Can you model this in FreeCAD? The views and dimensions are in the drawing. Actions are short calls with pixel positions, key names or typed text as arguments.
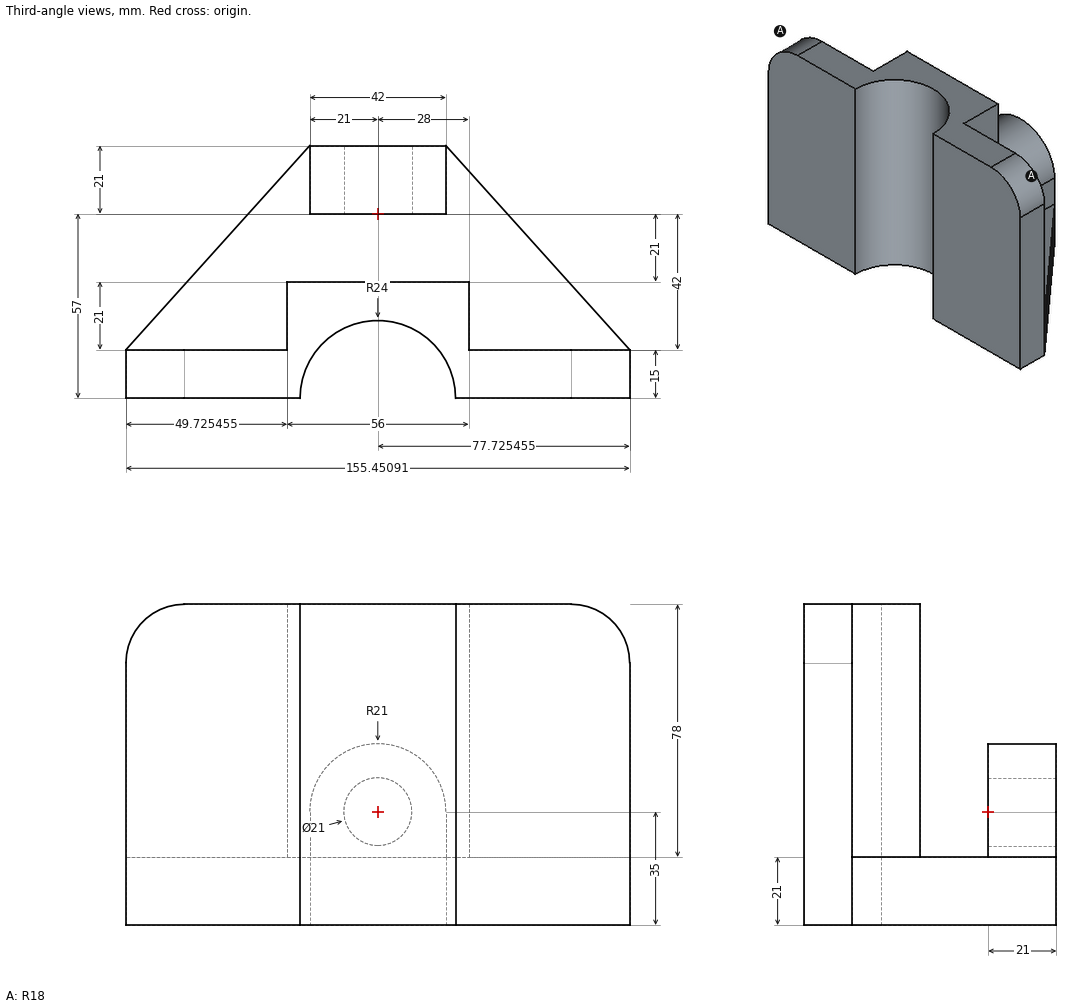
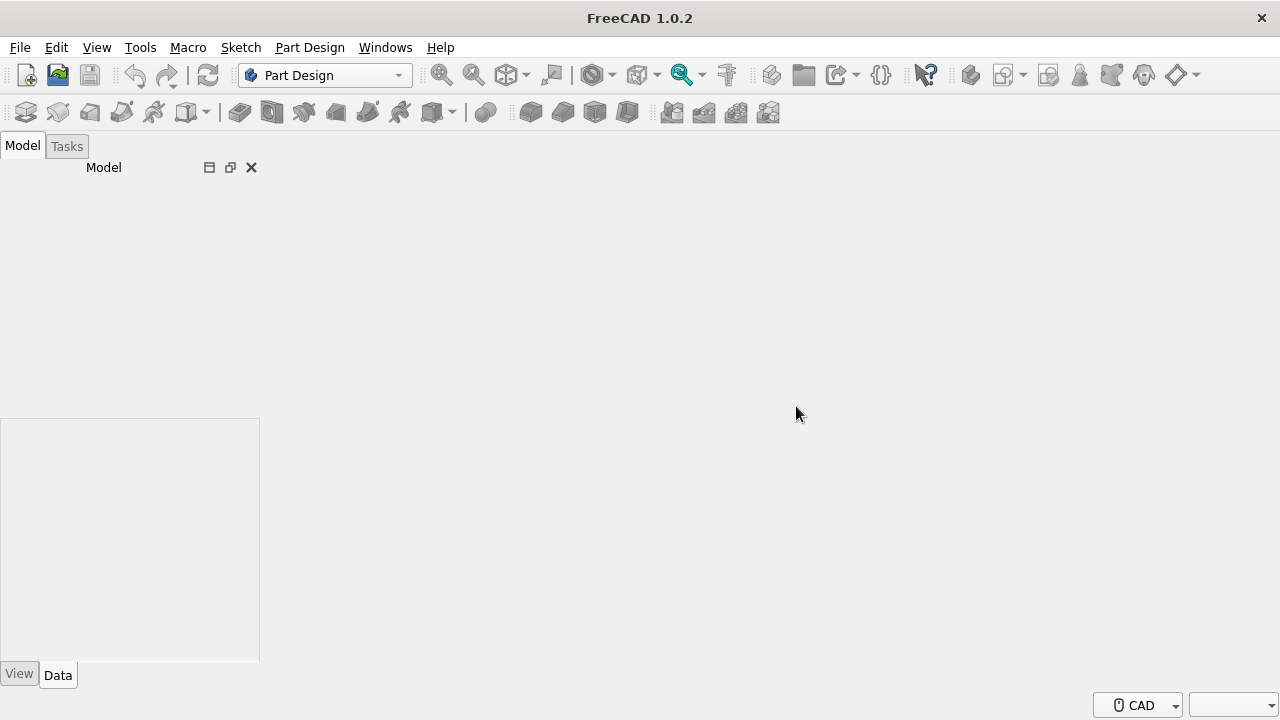
click(26, 76)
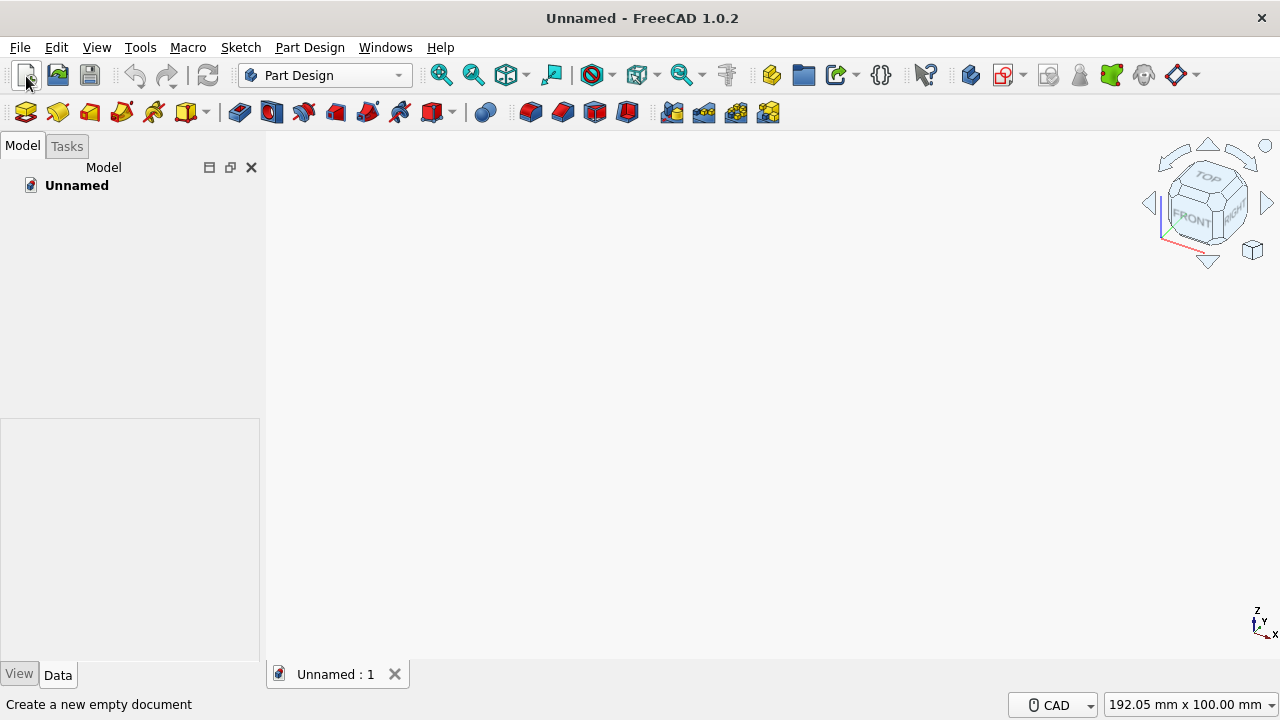
click(1004, 76)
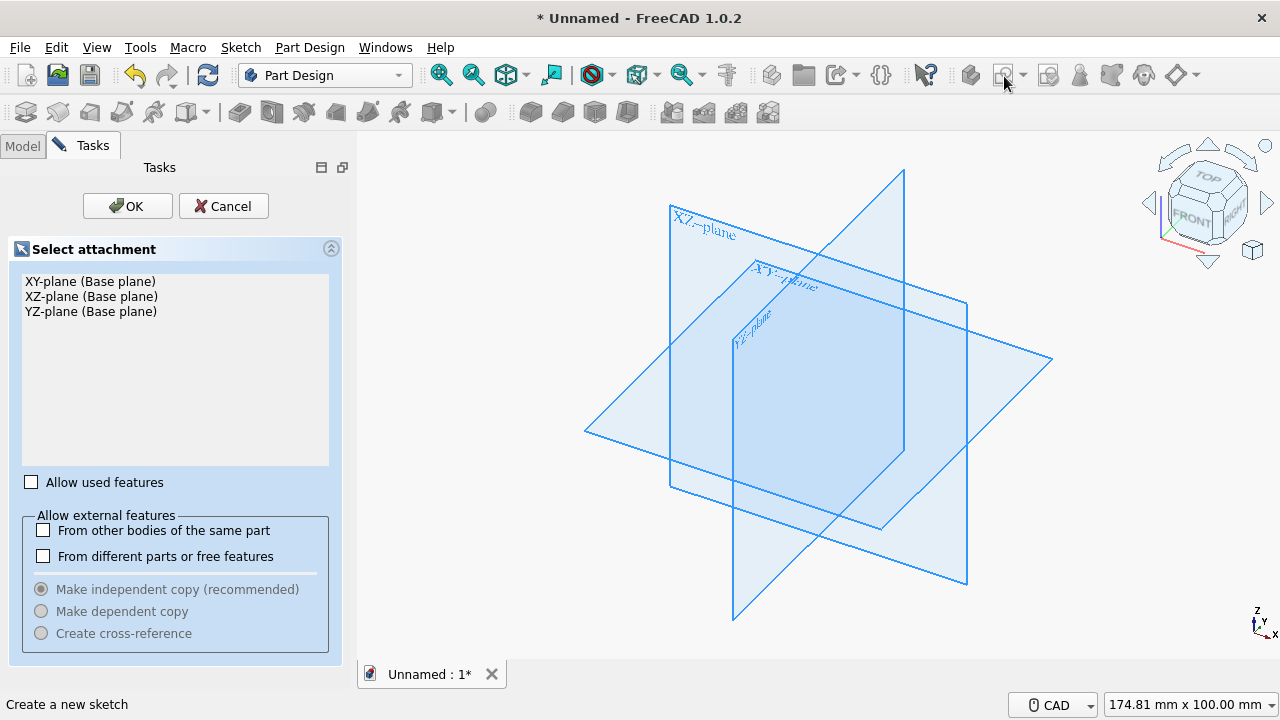
click(82, 296)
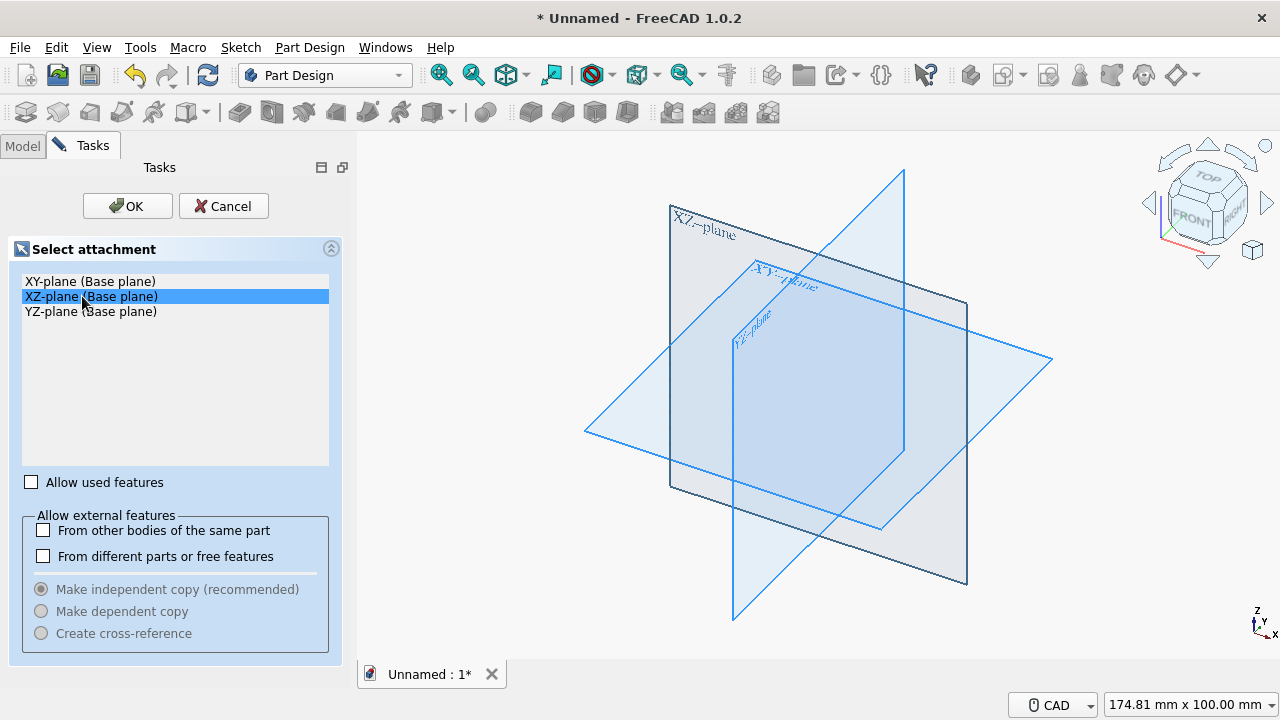
click(128, 206)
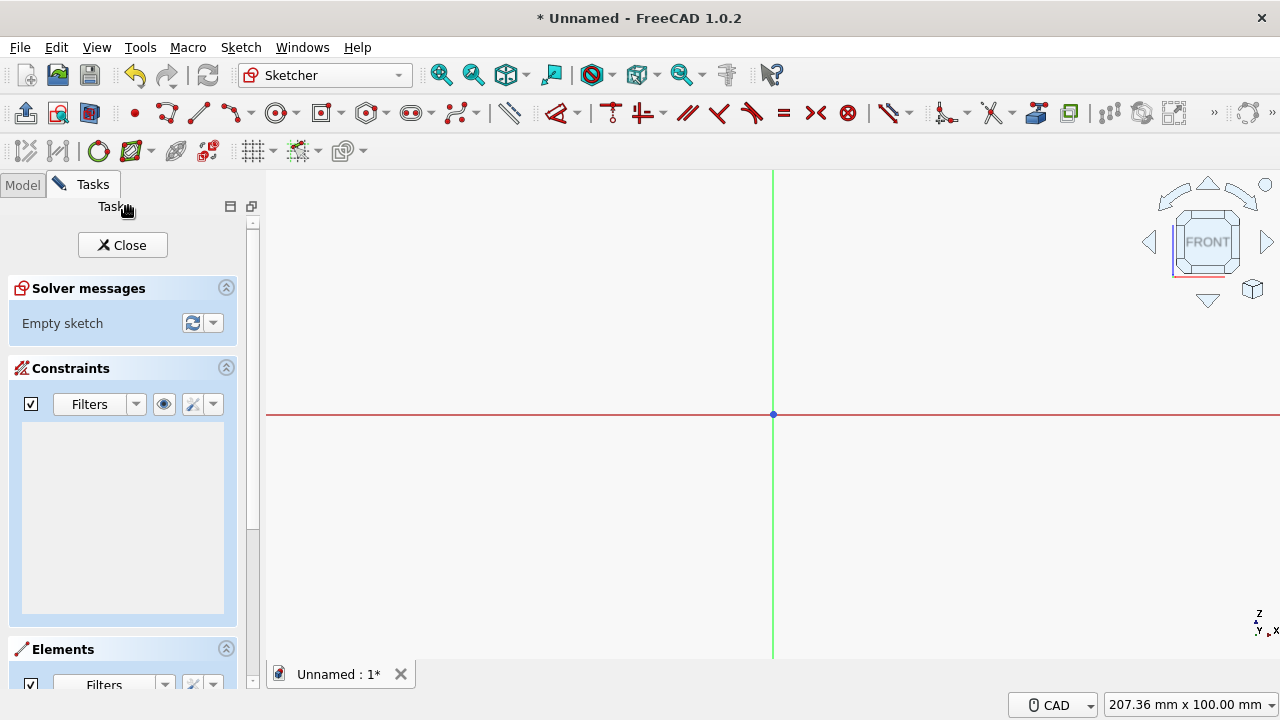
click(168, 114)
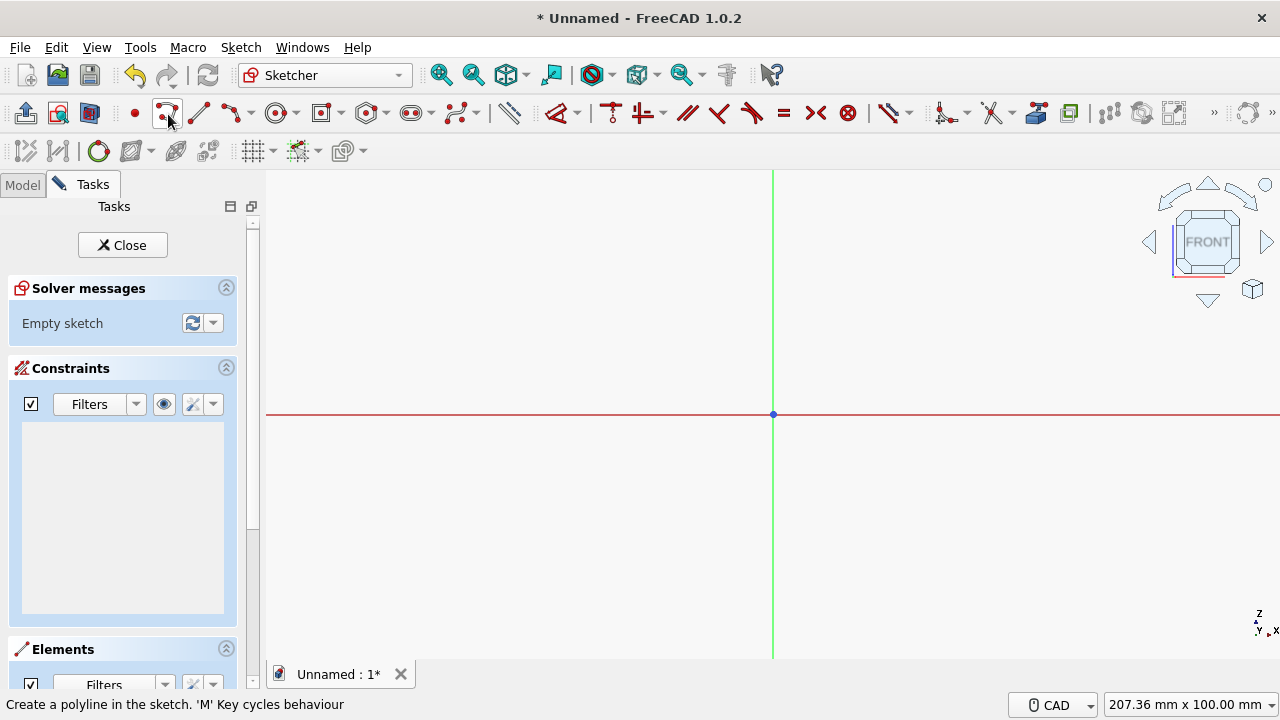
click(876, 414)
click(876, 586)
click(670, 586)
click(670, 414)
right_click(670, 414)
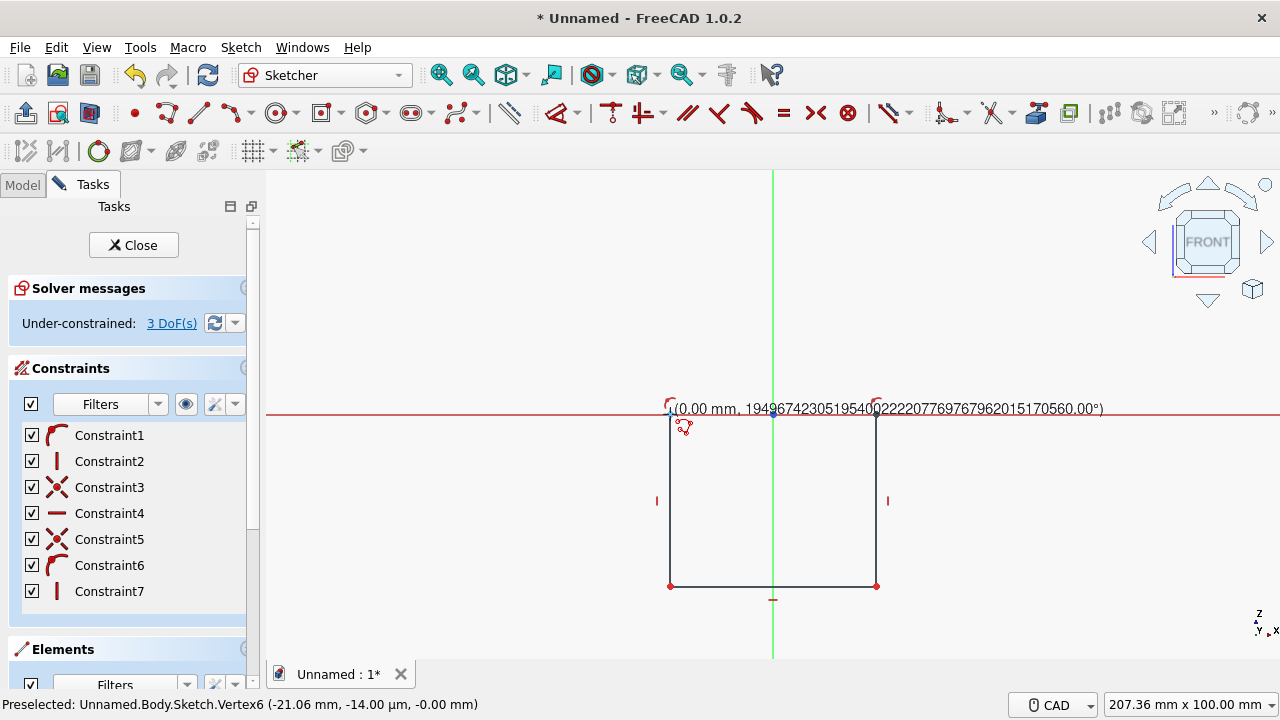
click(232, 114)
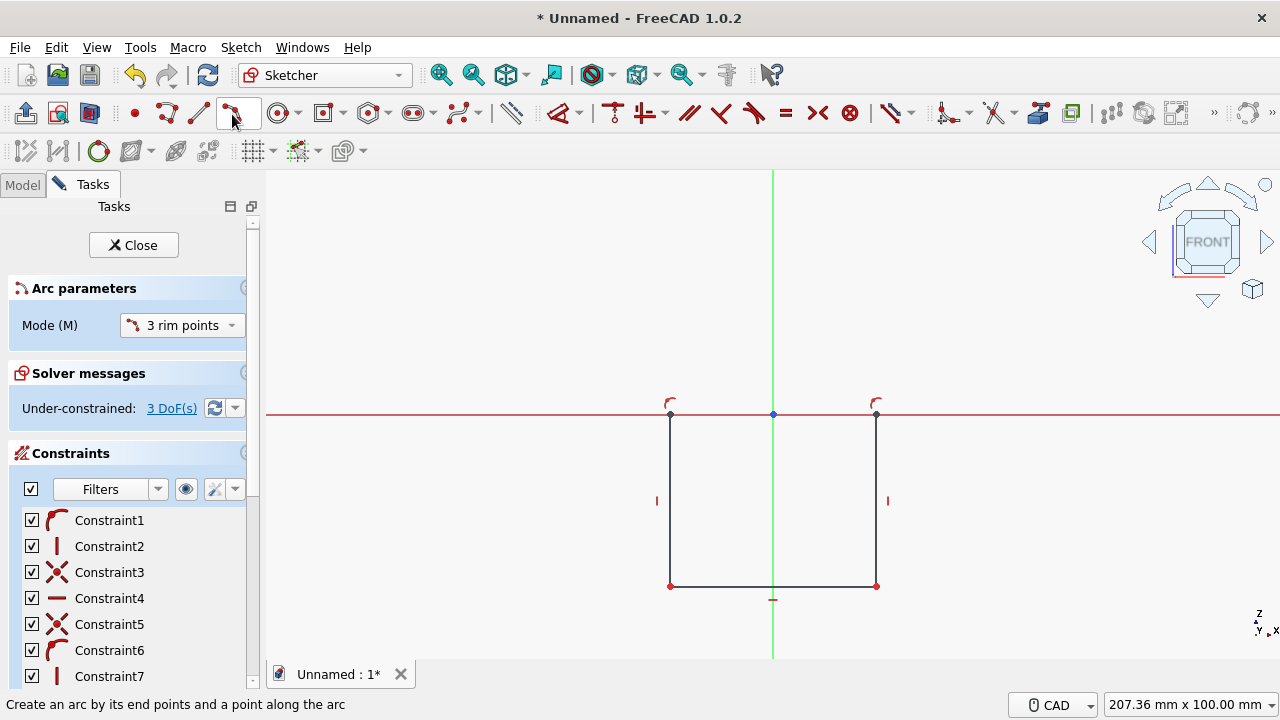
click(670, 414)
click(876, 414)
click(805, 317)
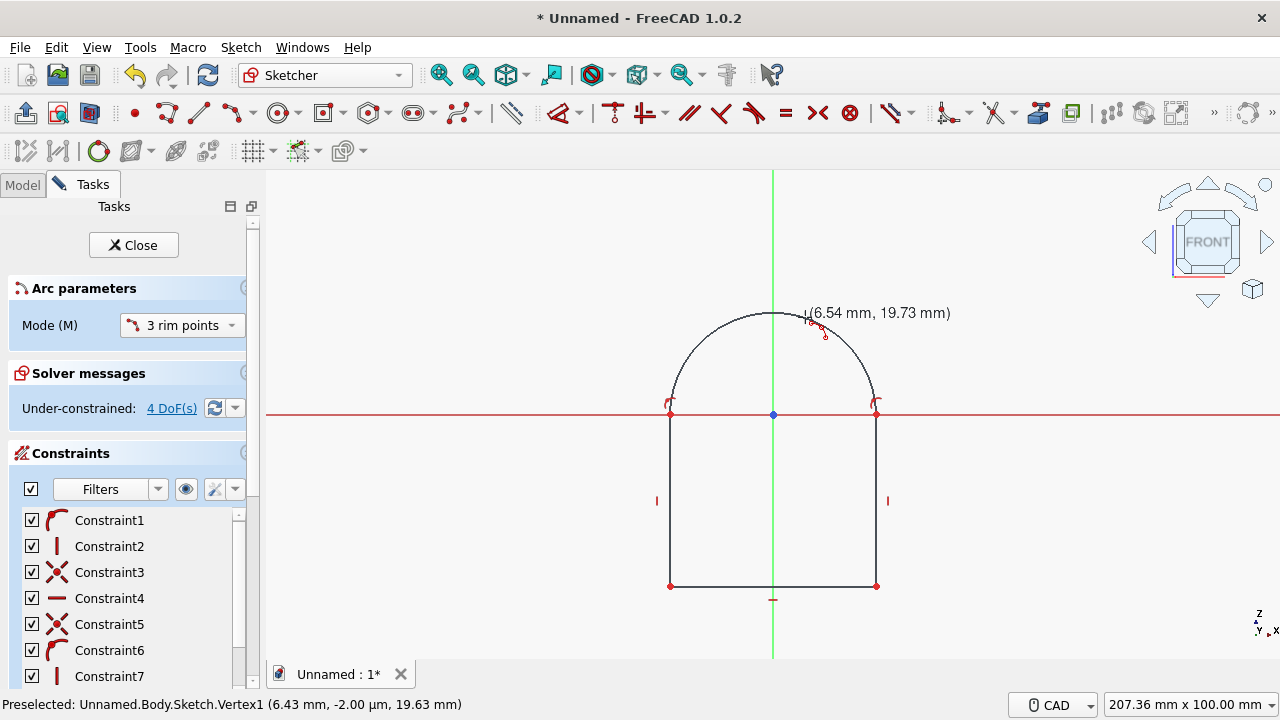
key(g)
key(c)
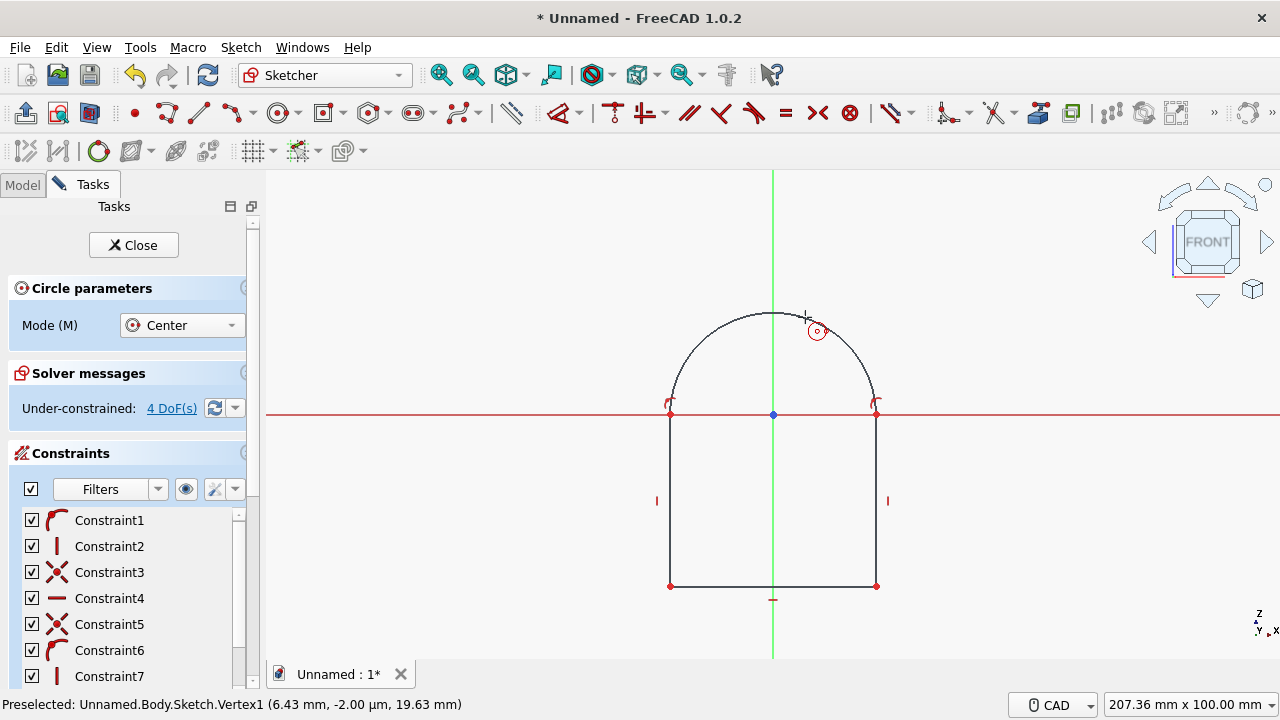
click(773, 414)
move(809, 378)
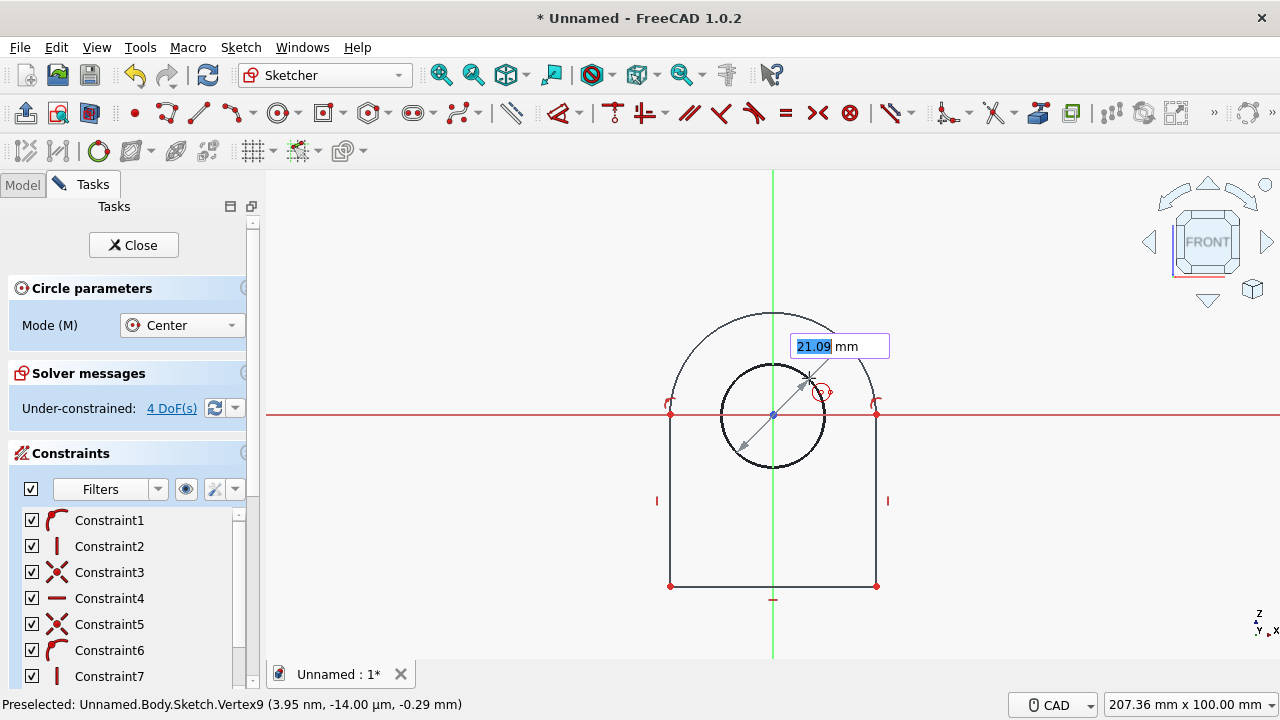
text(21)
key(Return)
key(Escape)